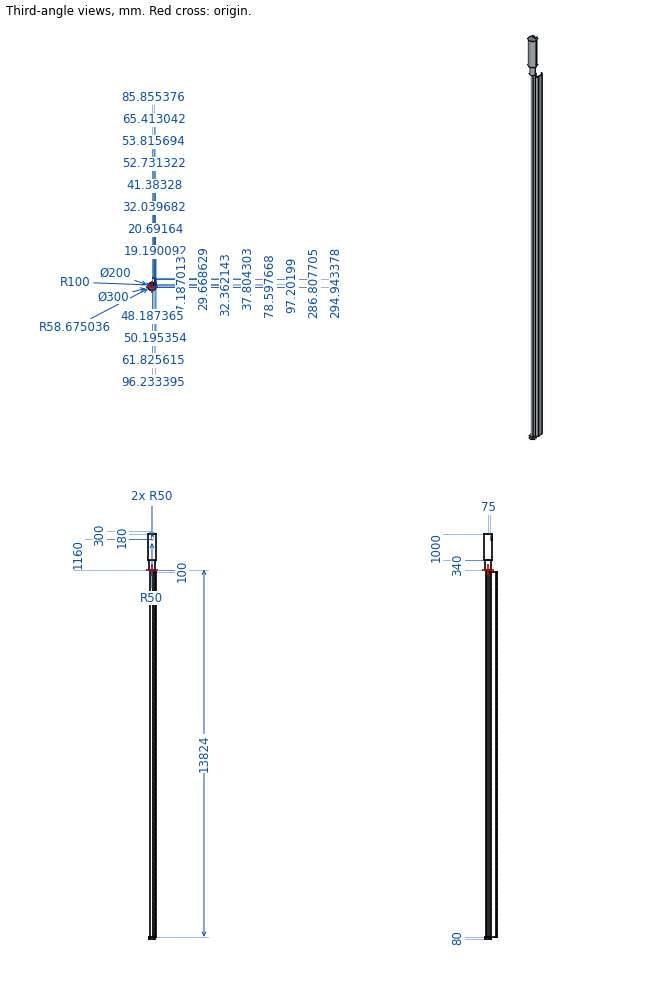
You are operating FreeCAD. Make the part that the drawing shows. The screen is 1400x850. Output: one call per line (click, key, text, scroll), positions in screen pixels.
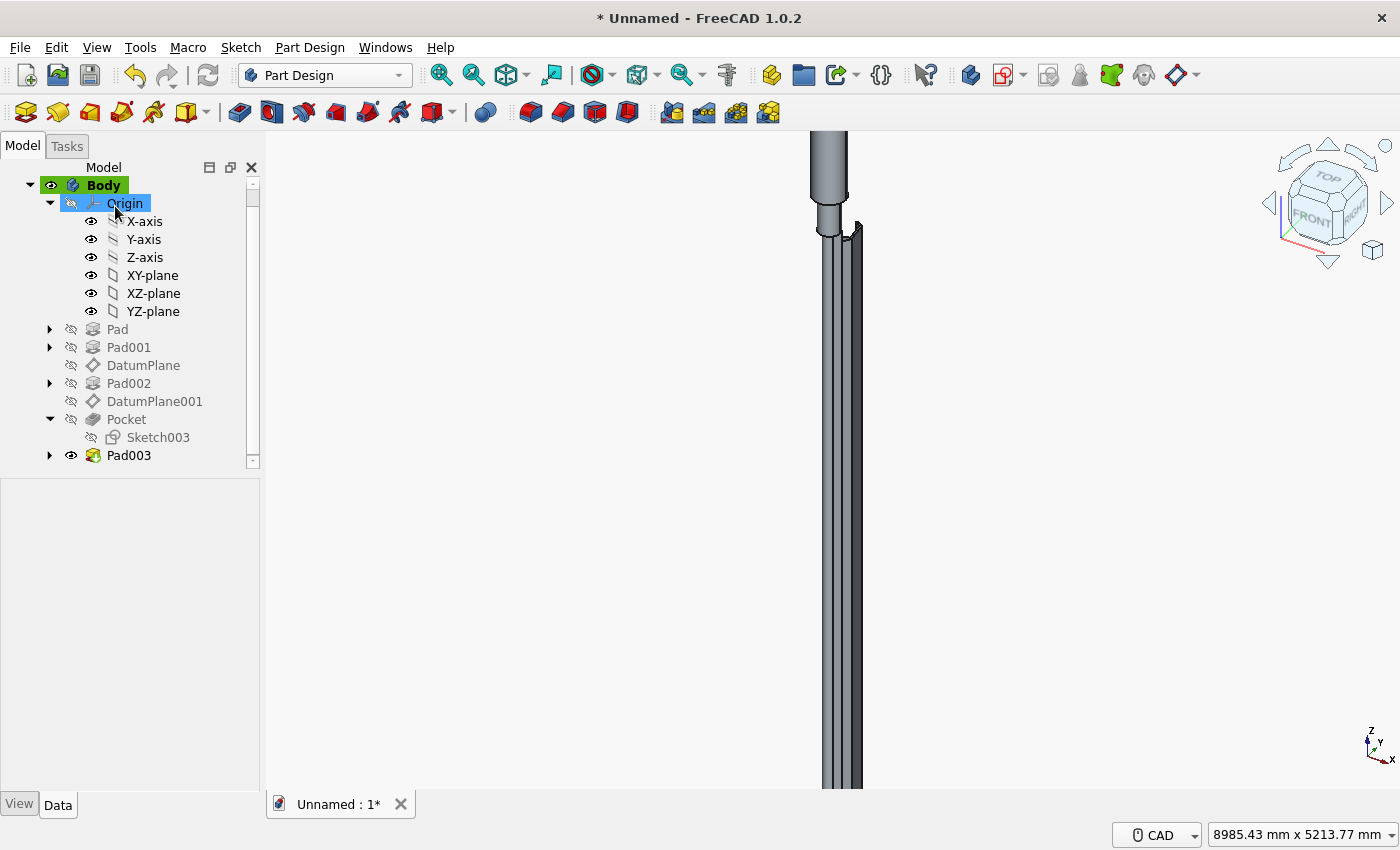
click(442, 76)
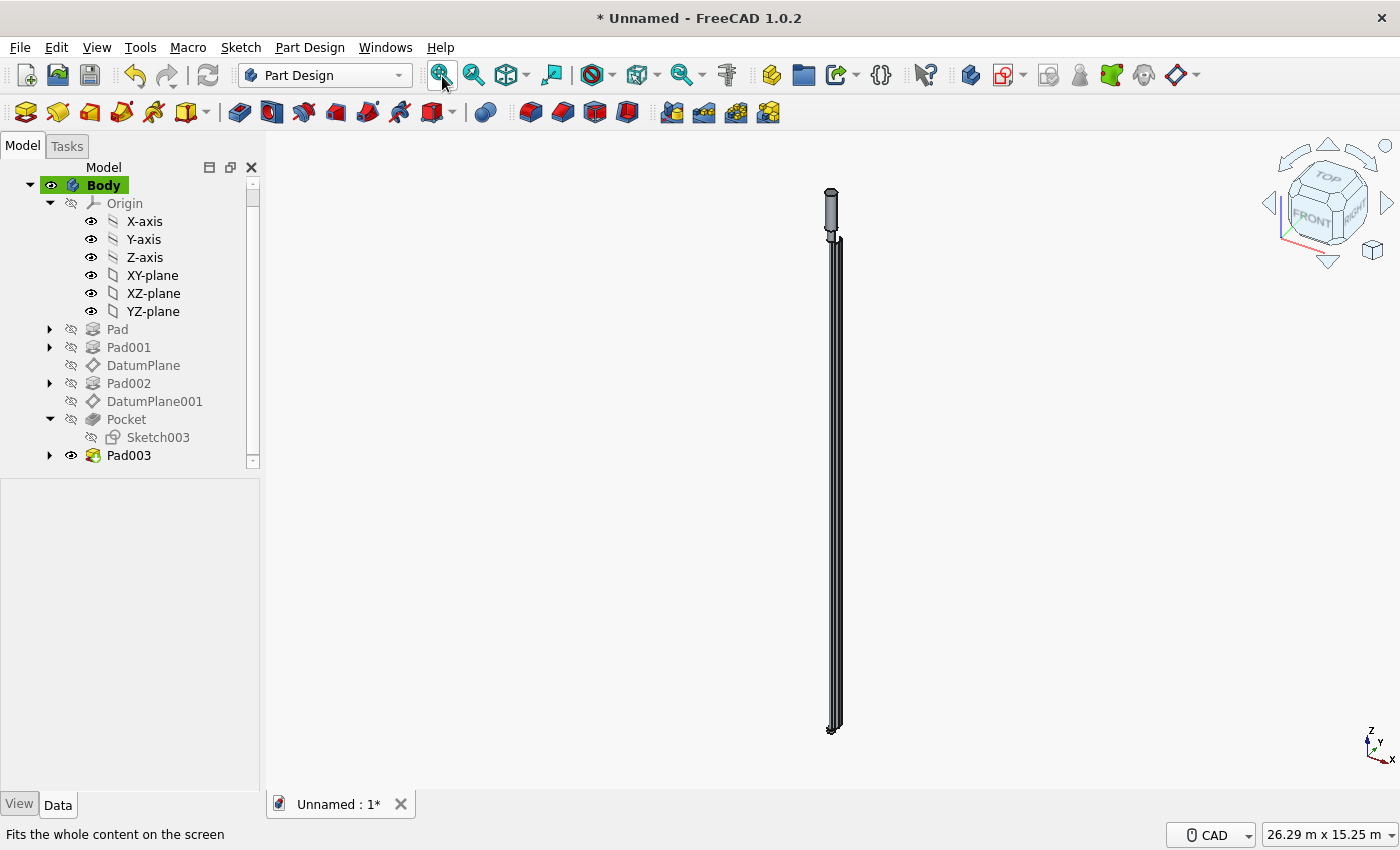
click(1004, 76)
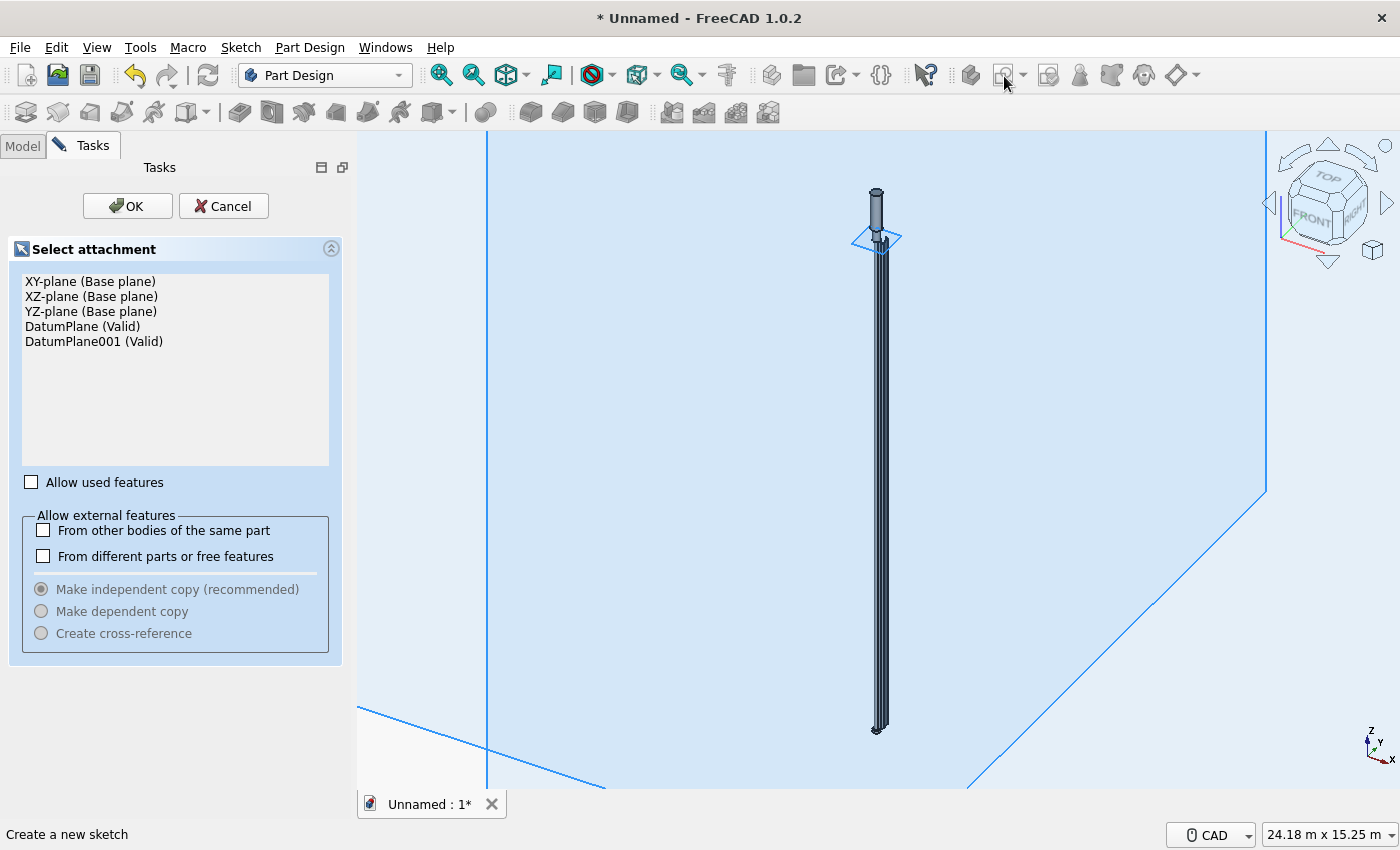
click(82, 296)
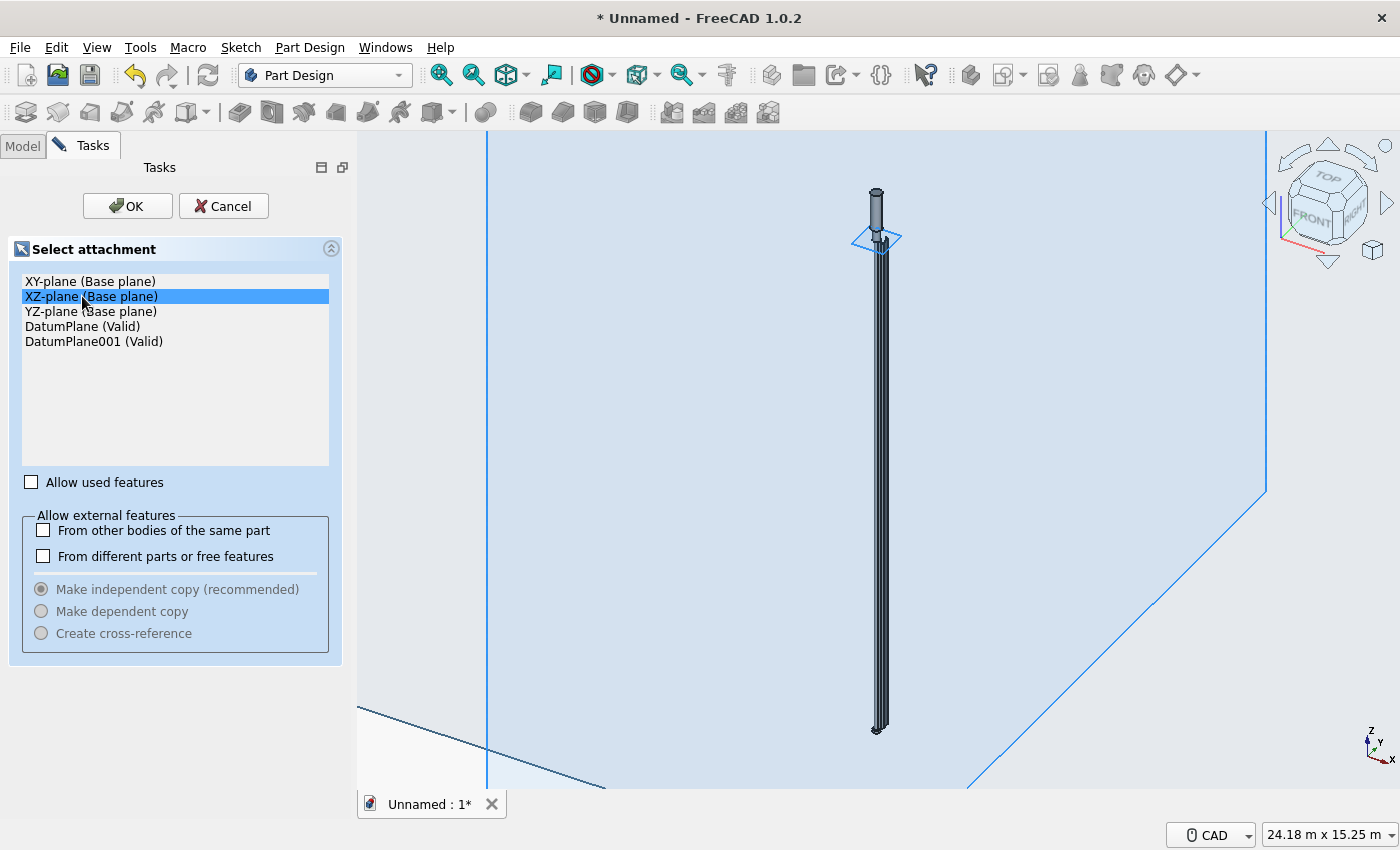
click(128, 206)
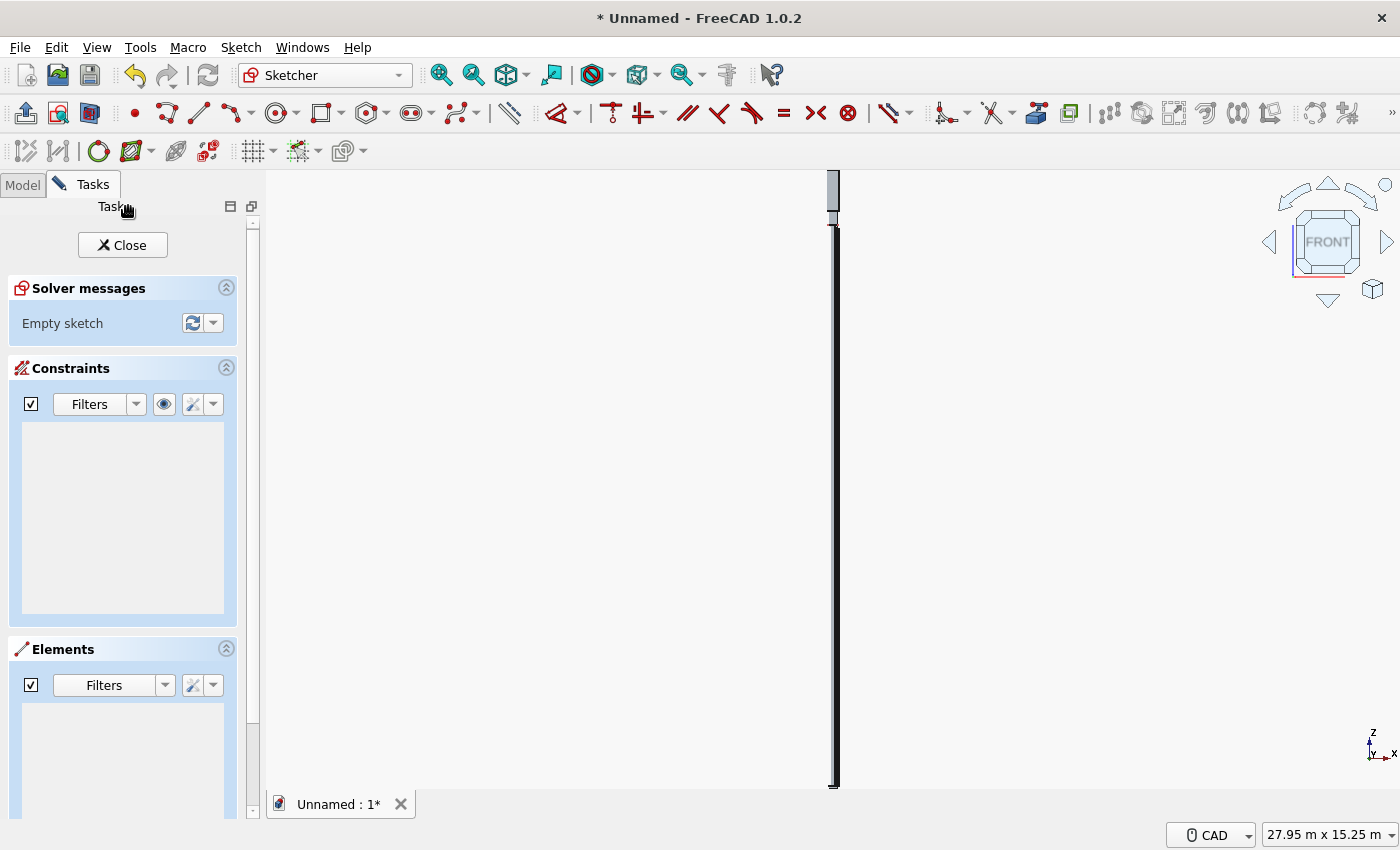
key(q)
key(s)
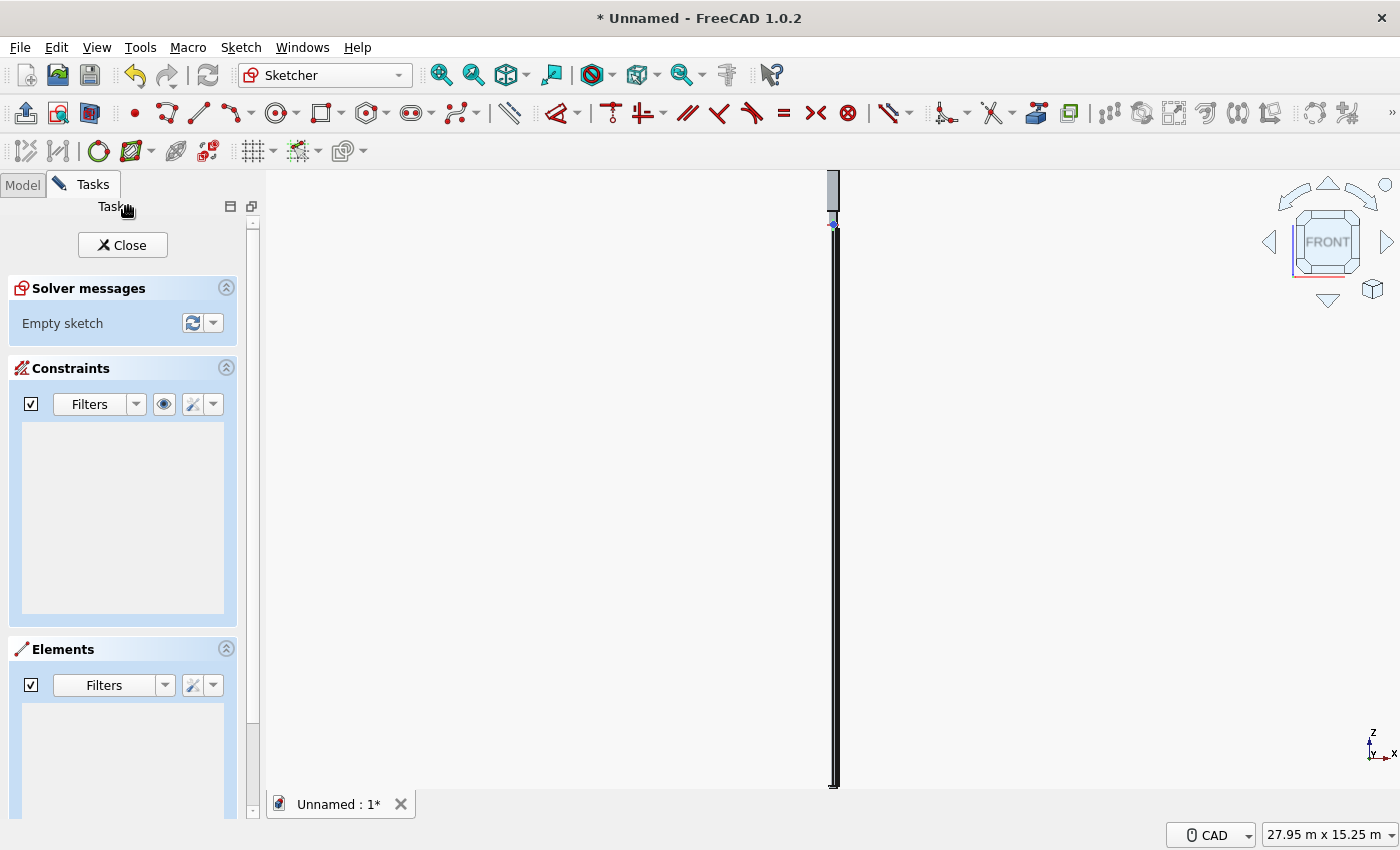
scroll(764, 480, down, 5)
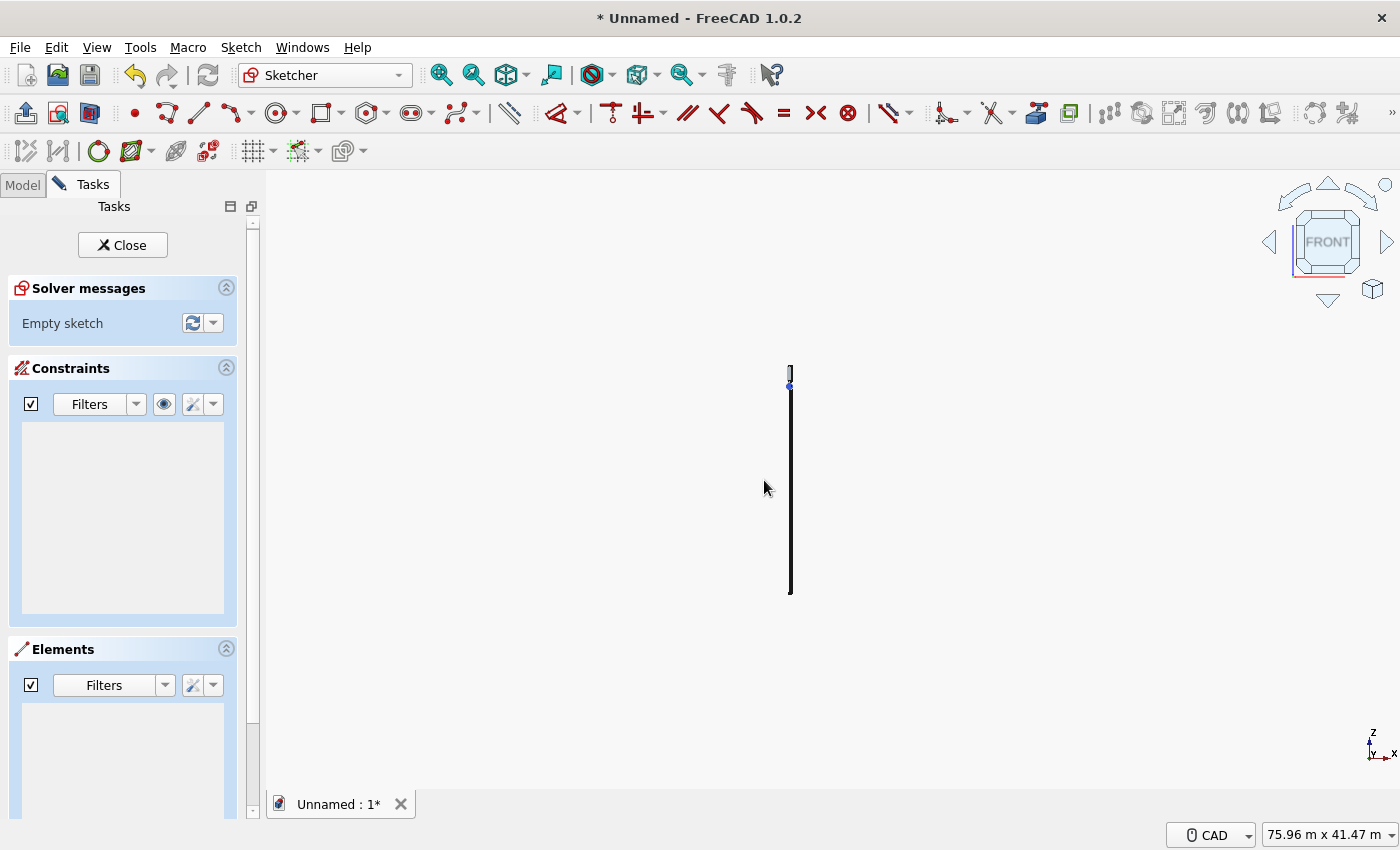
scroll(791, 361, up, 15)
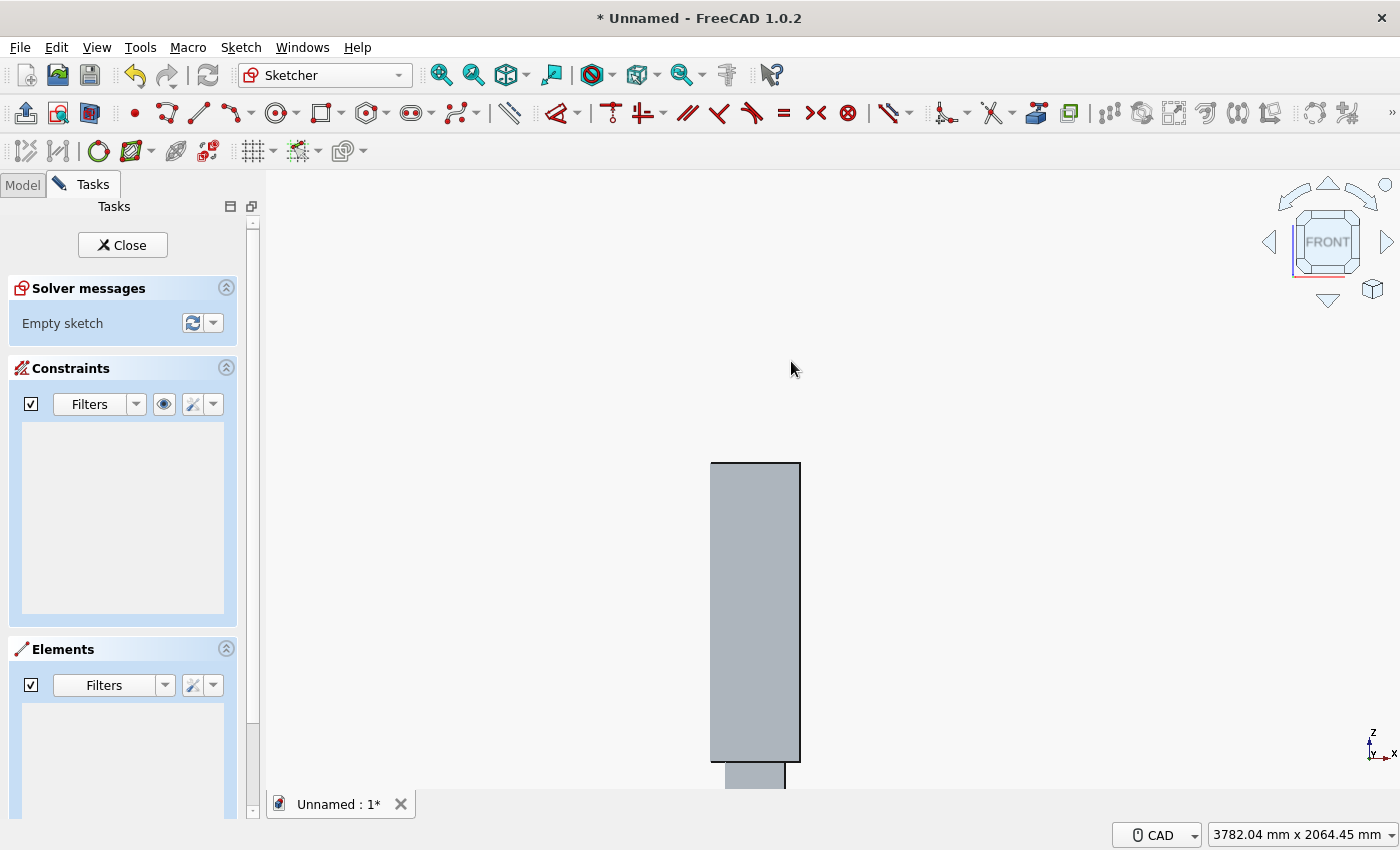
scroll(751, 468, up, 6)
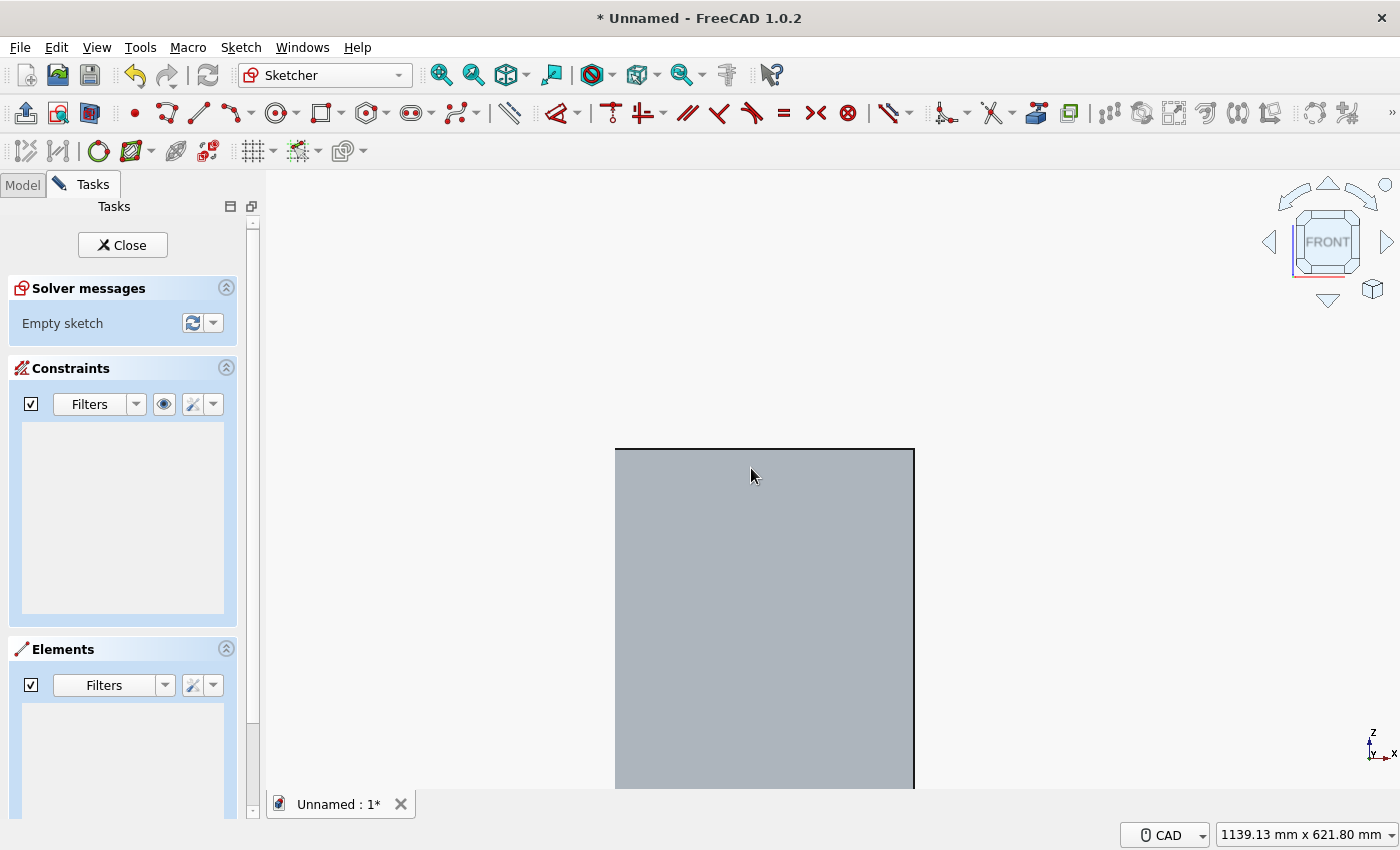
key(g)
key(s)